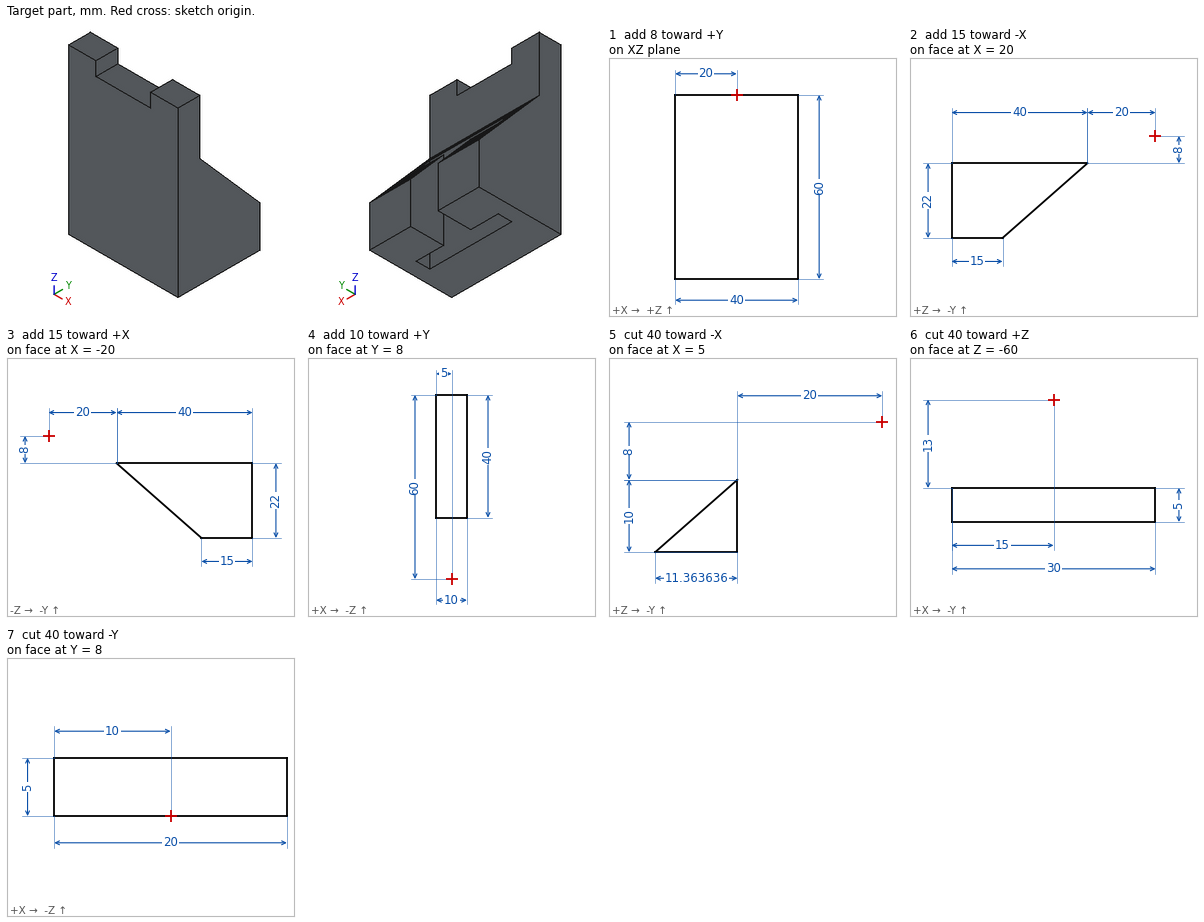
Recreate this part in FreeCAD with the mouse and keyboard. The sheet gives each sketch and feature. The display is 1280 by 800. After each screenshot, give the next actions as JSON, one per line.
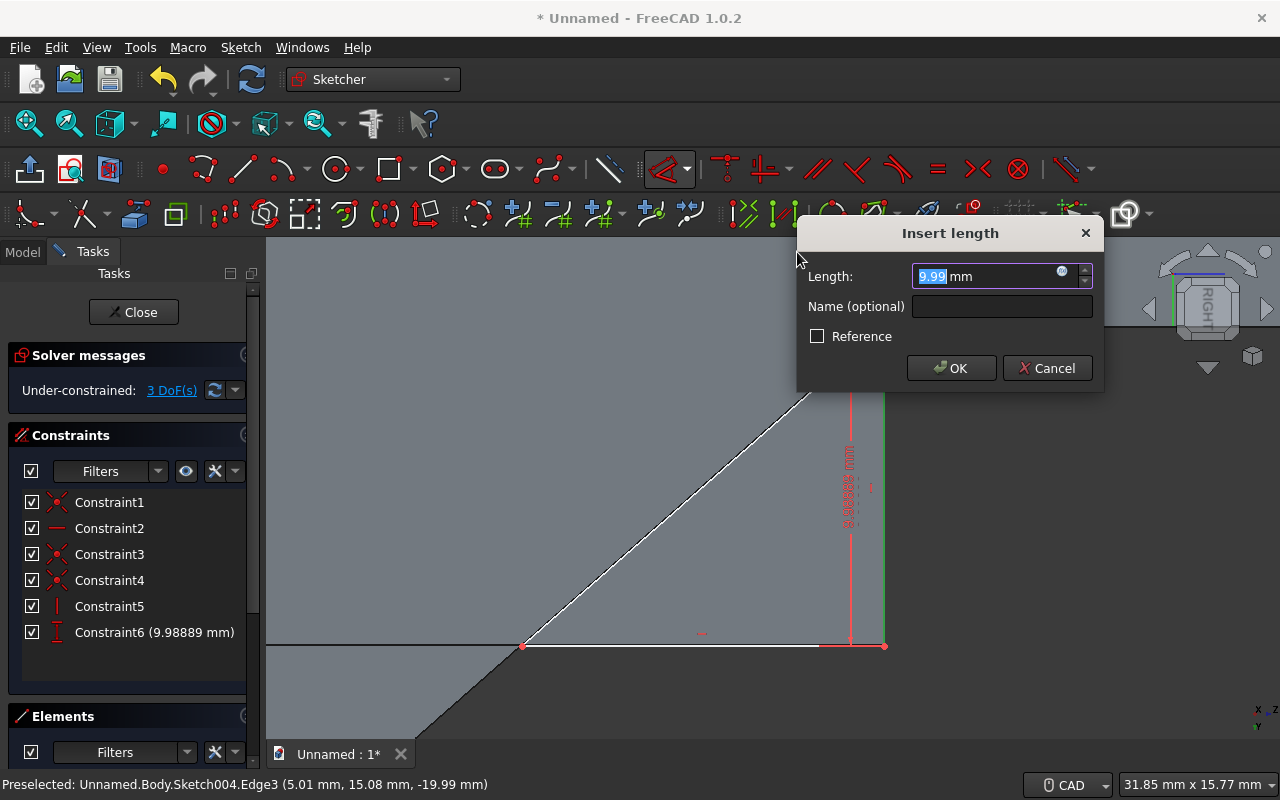
{"action": "type", "text": "10"}
{"action": "key", "text": "Return"}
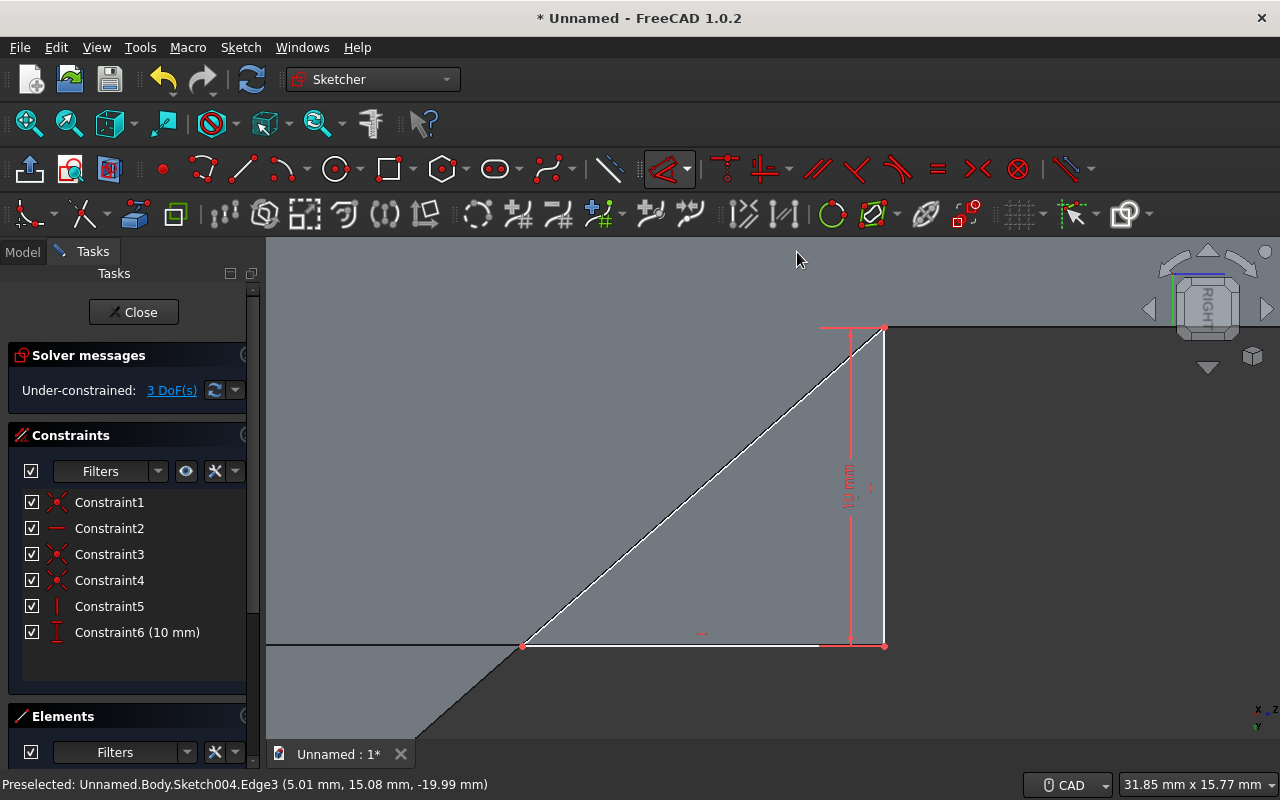
{"action": "left_click", "coordinate": [884, 328]}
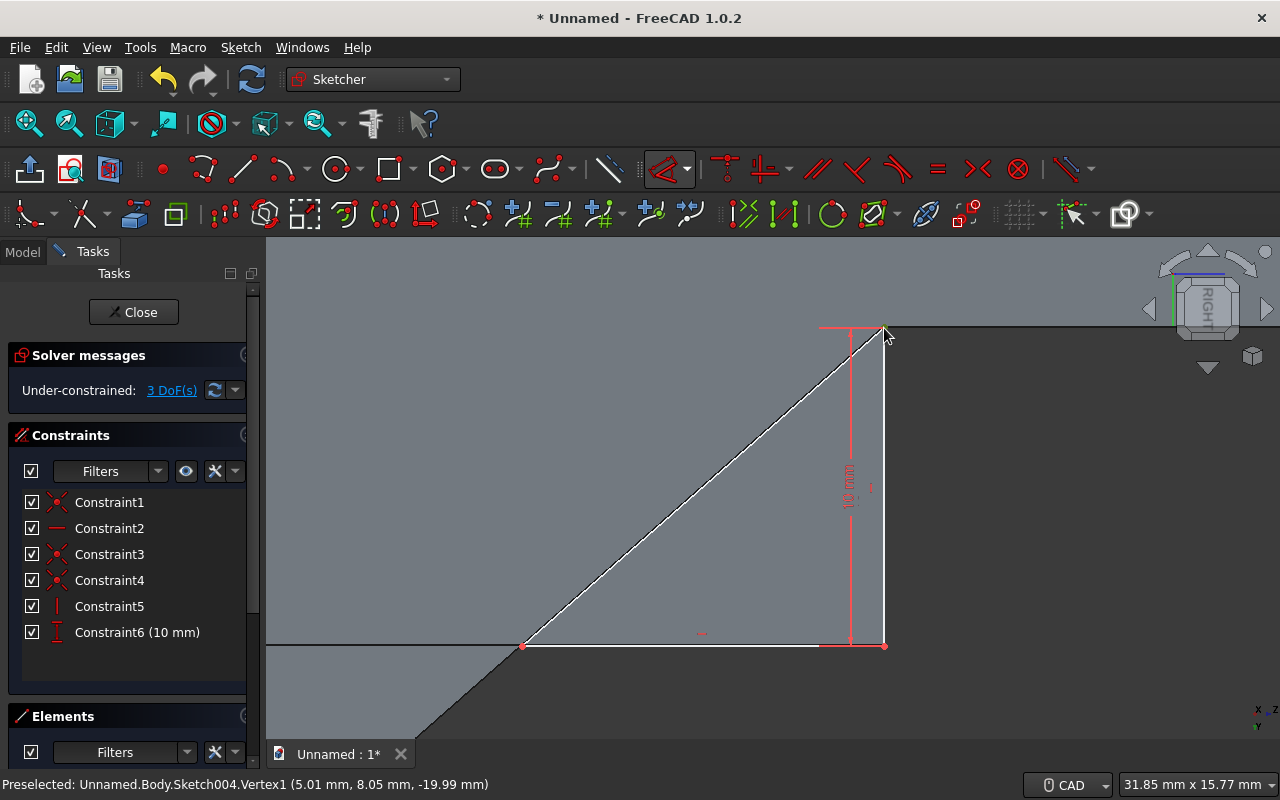
{"action": "left_click", "coordinate": [690, 170]}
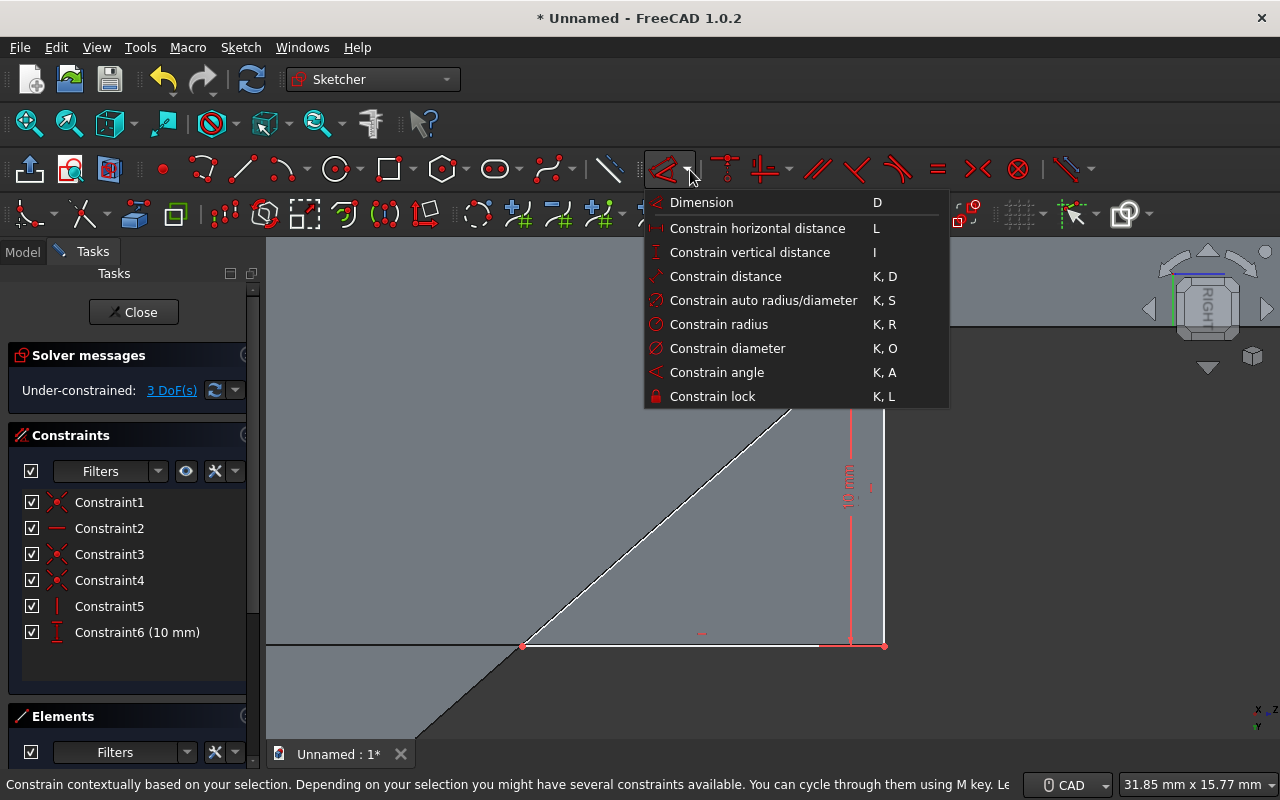
{"action": "left_click", "coordinate": [797, 252]}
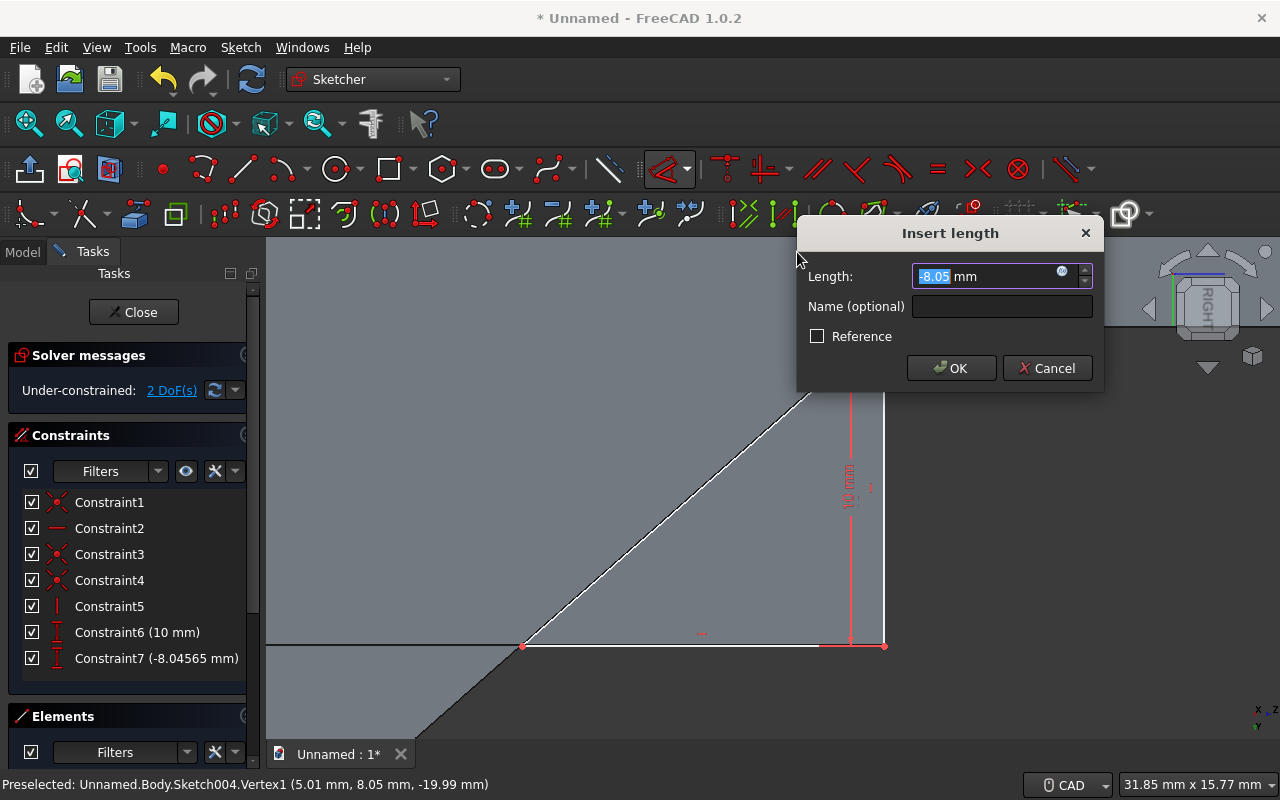
{"action": "type", "text": "-8"}
{"action": "key", "text": "Return"}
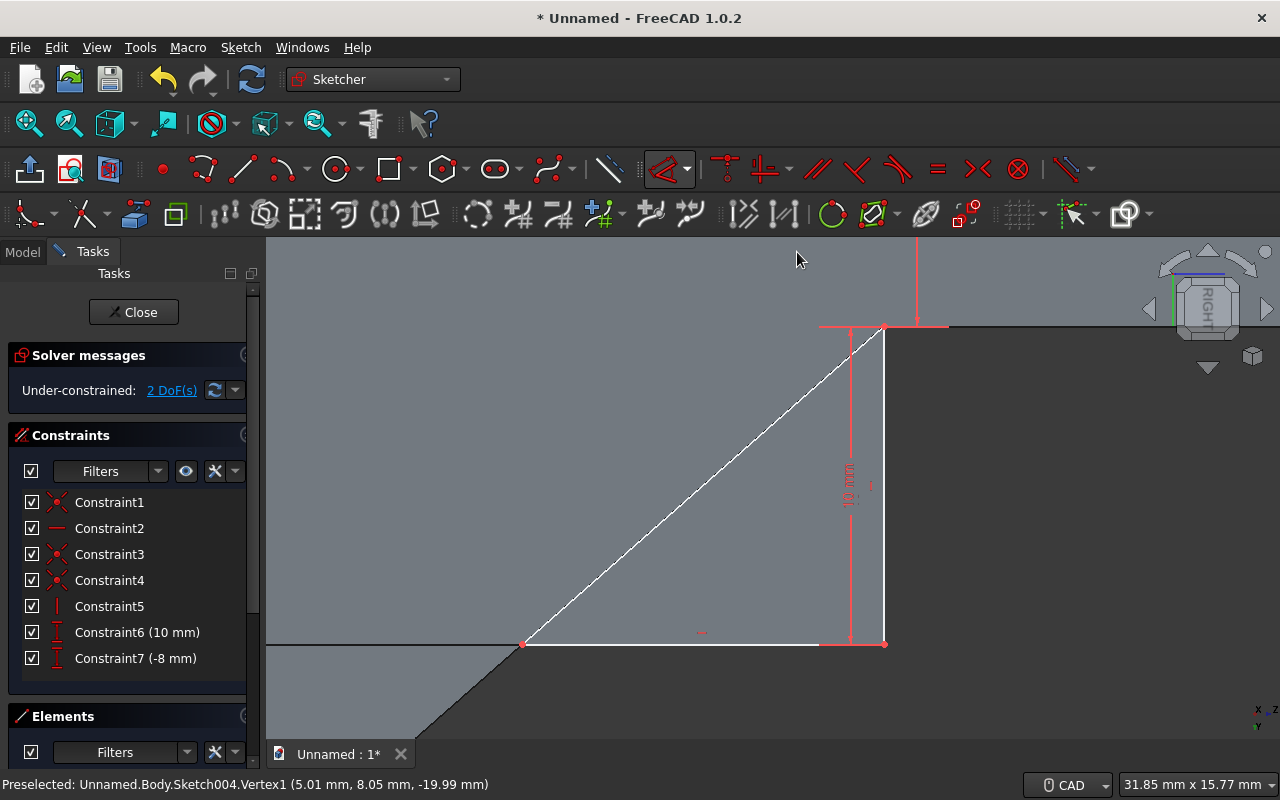
{"action": "left_click", "coordinate": [884, 327]}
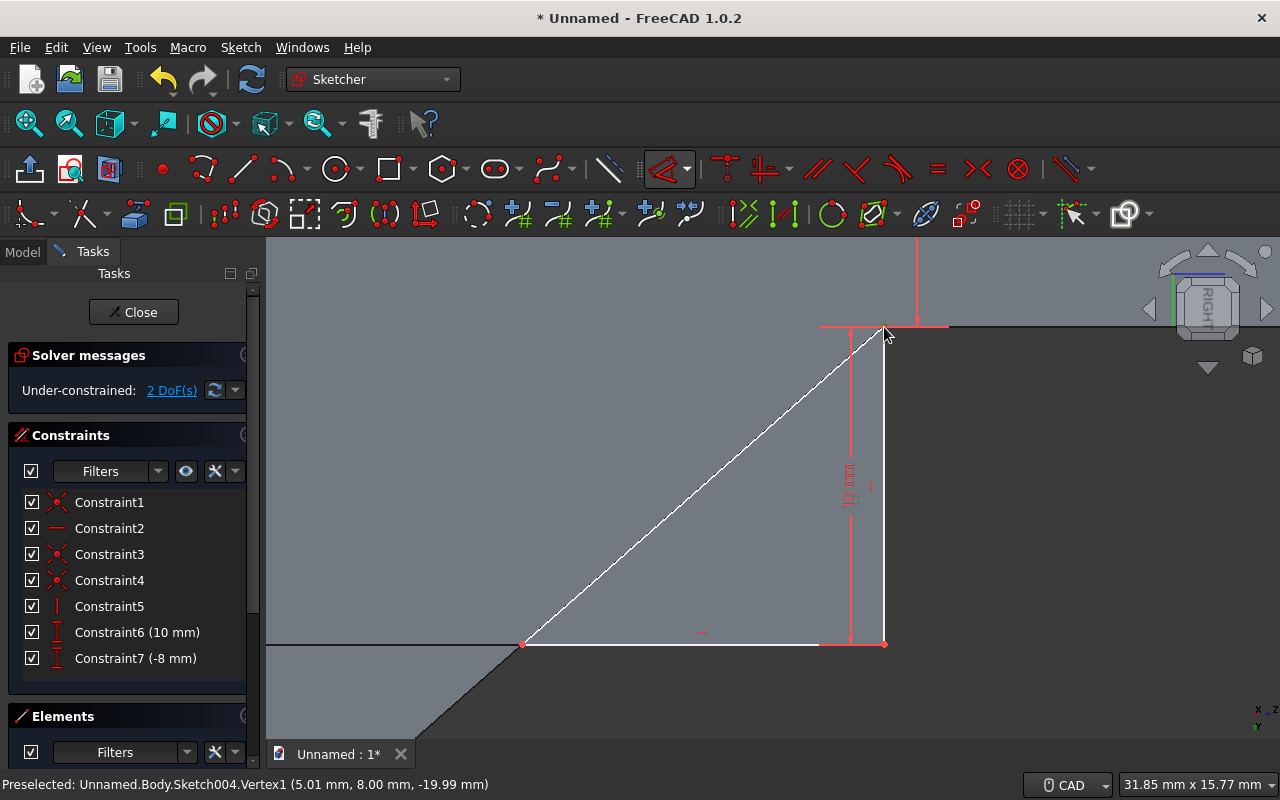
{"action": "key", "text": "l"}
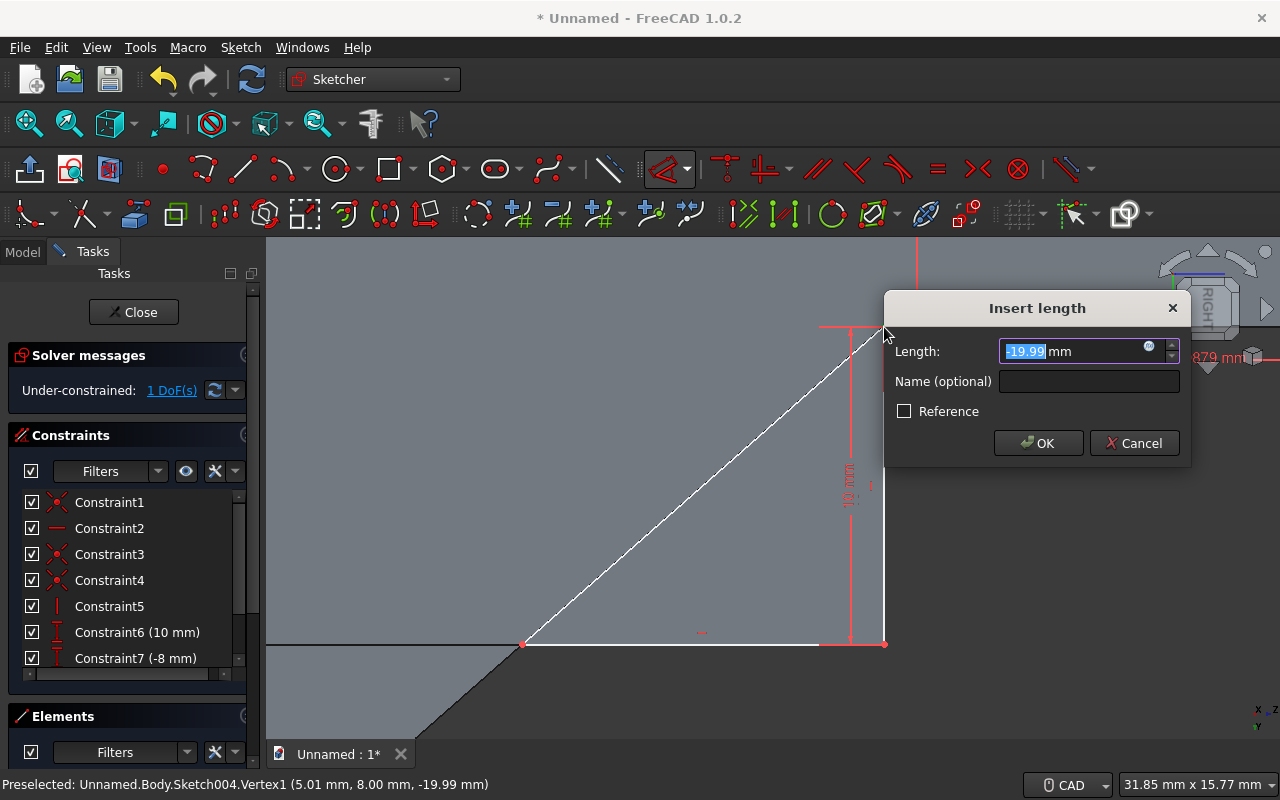
{"action": "type", "text": "-20"}
{"action": "key", "text": "Return"}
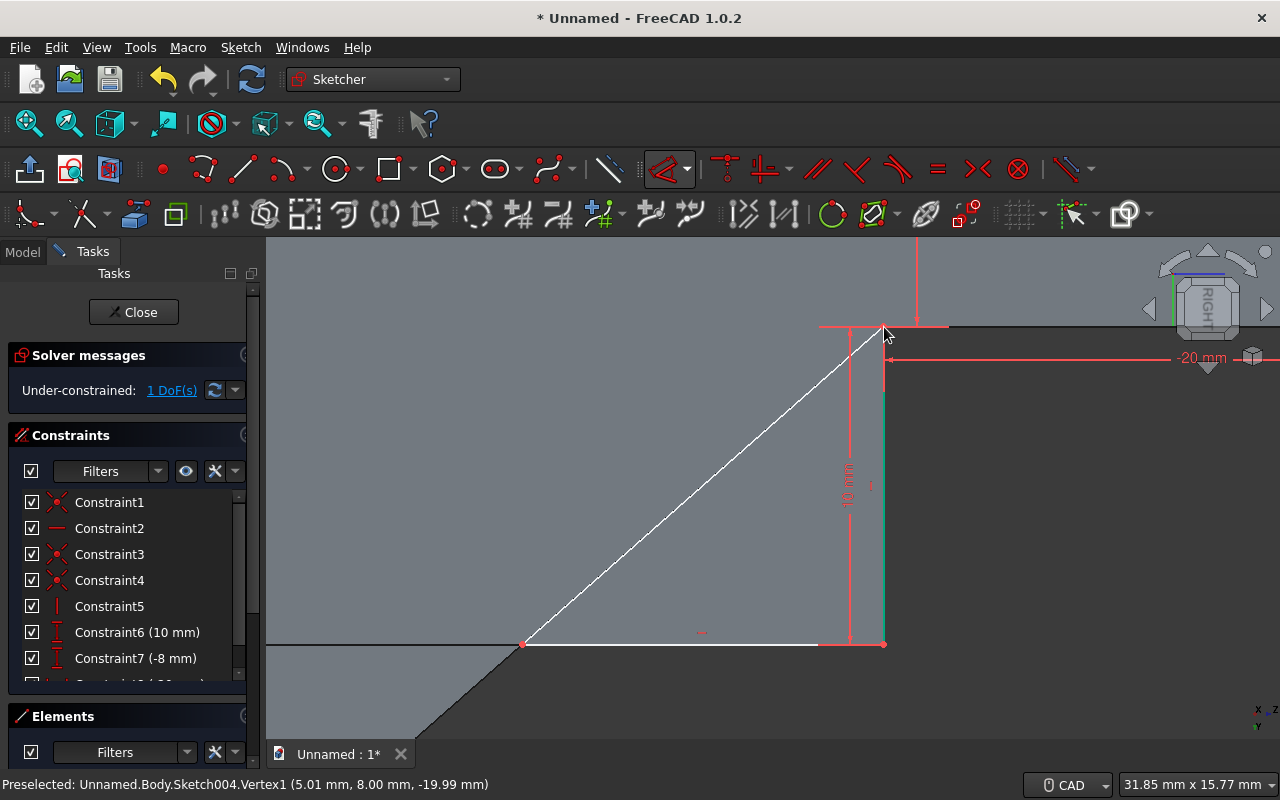
{"action": "left_click", "coordinate": [630, 645]}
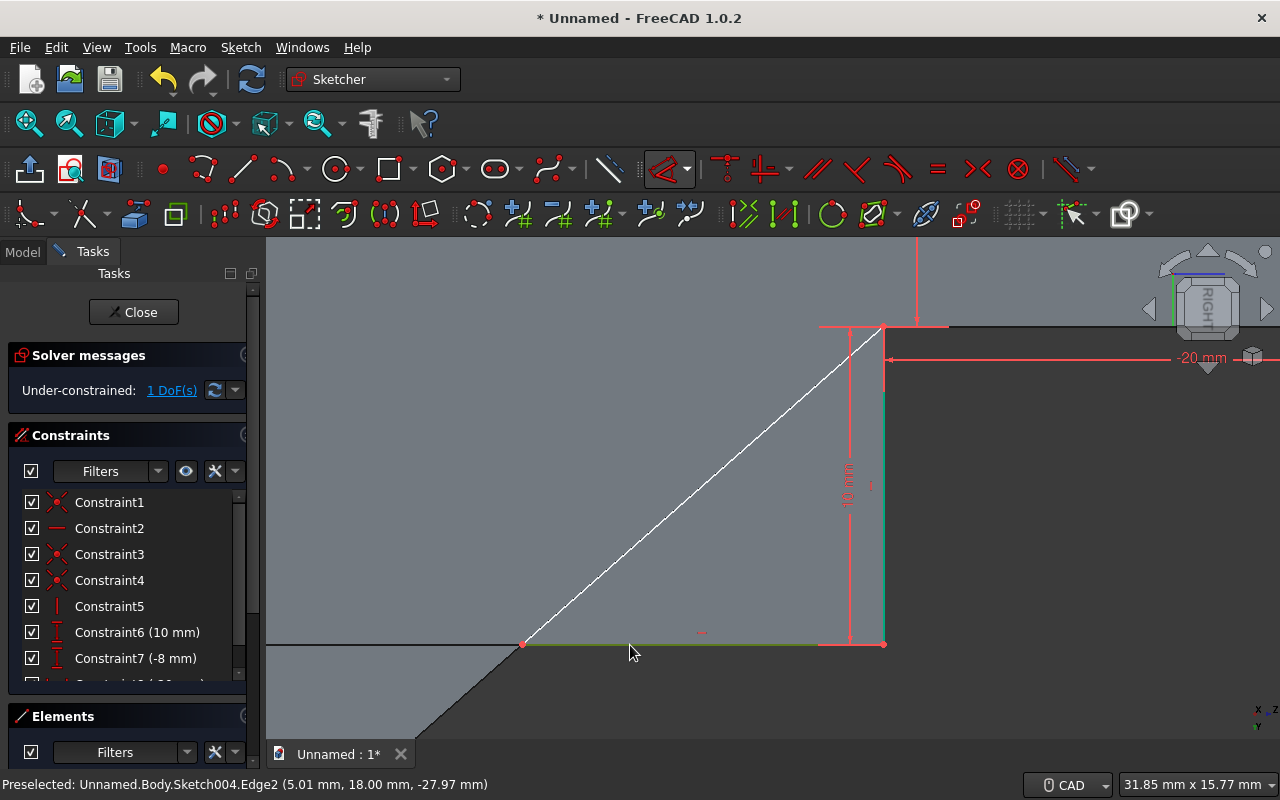
{"action": "key", "text": "l"}